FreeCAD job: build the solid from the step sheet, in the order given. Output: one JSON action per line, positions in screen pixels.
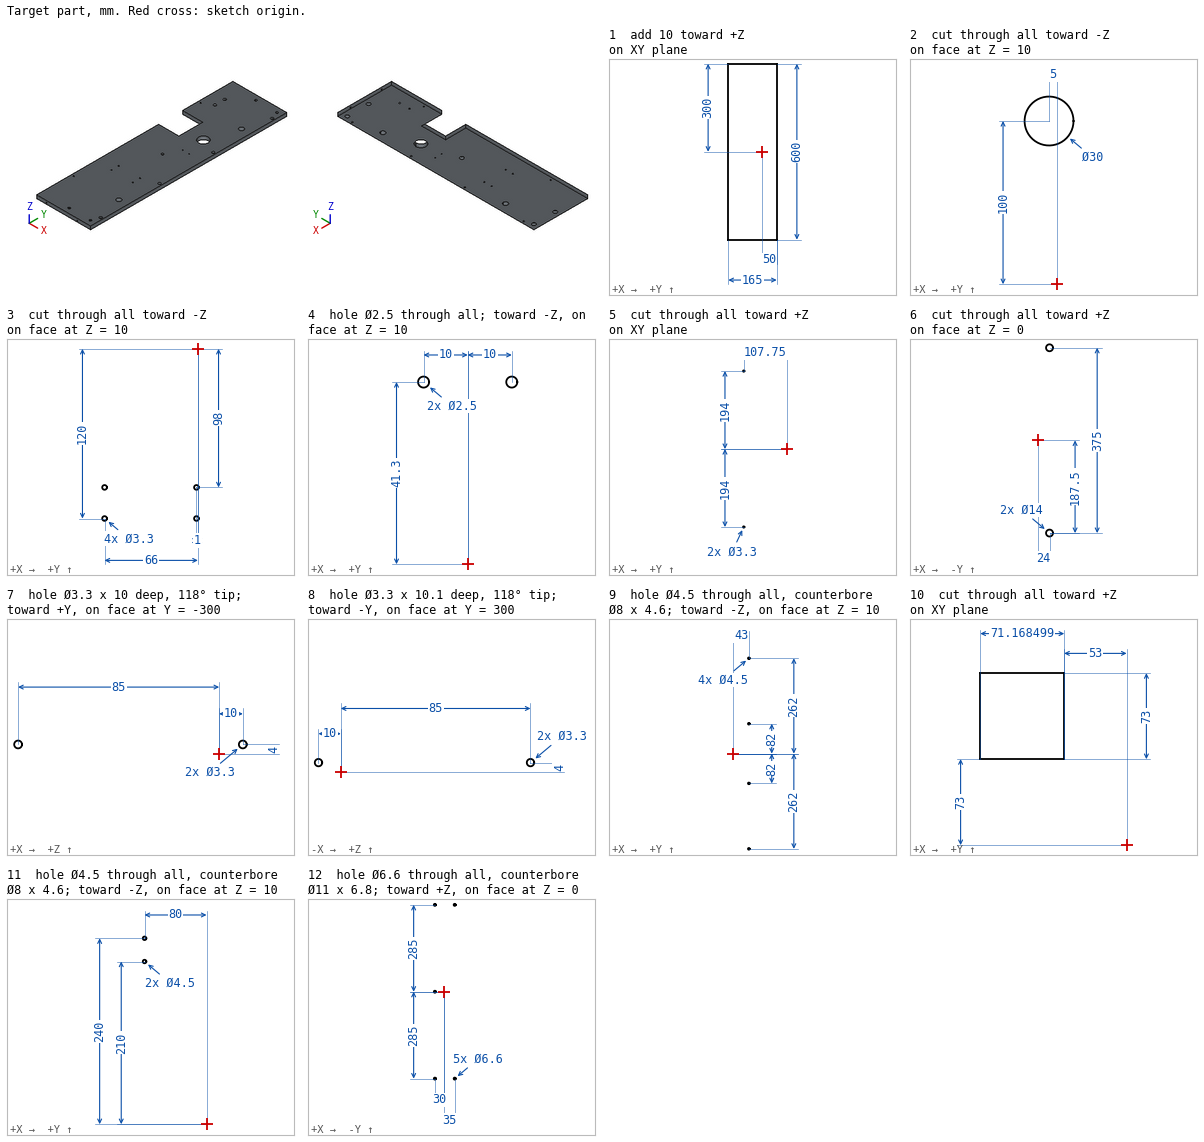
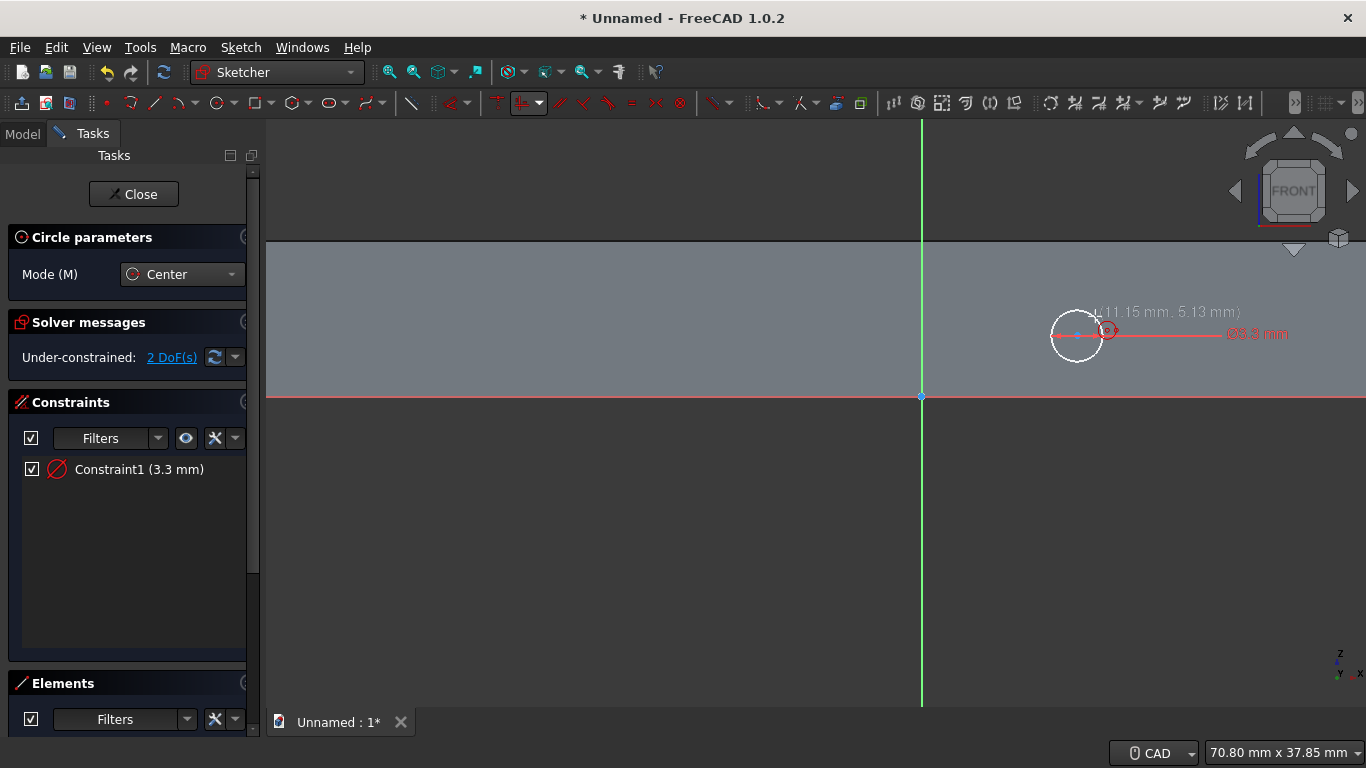
{"action": "scroll", "coordinate": [1081, 462], "scroll_direction": "down", "scroll_amount": 4}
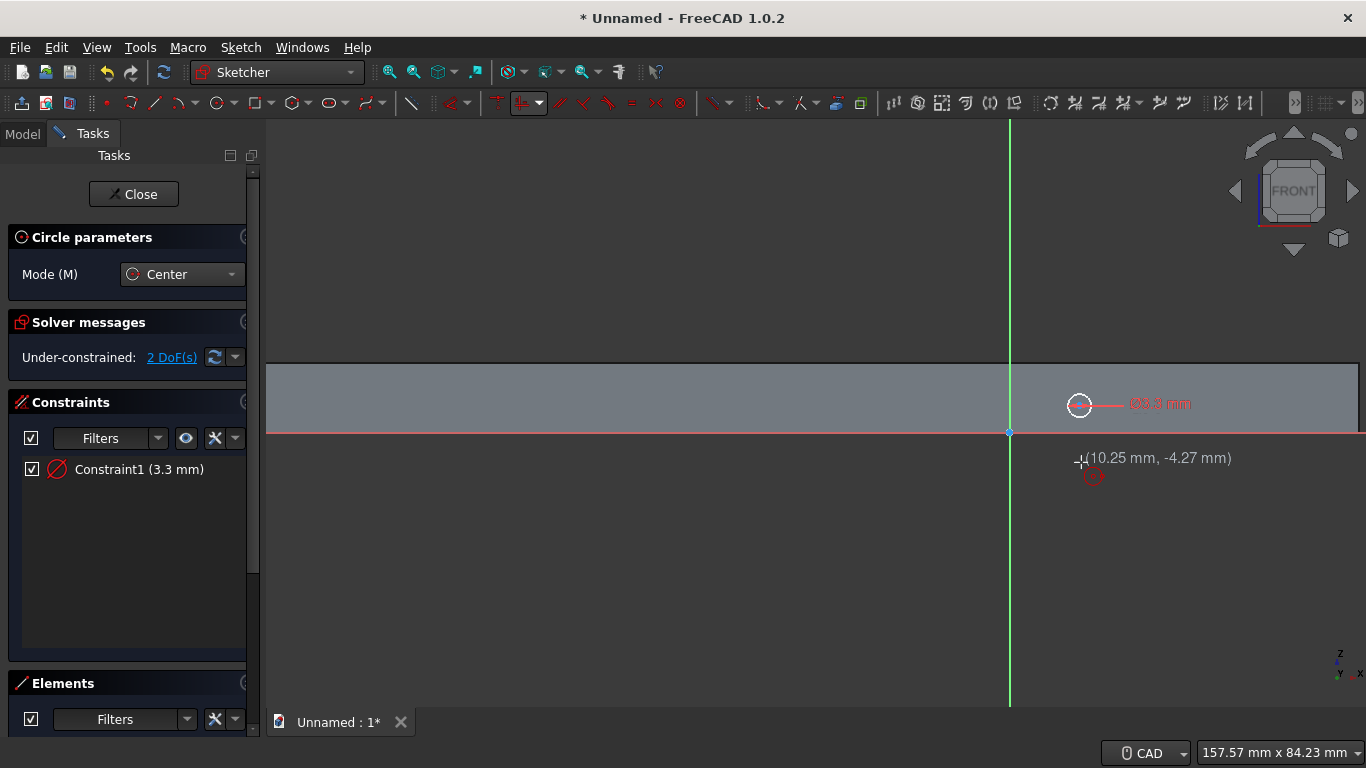
{"action": "scroll", "coordinate": [416, 405], "scroll_direction": "up", "scroll_amount": 4}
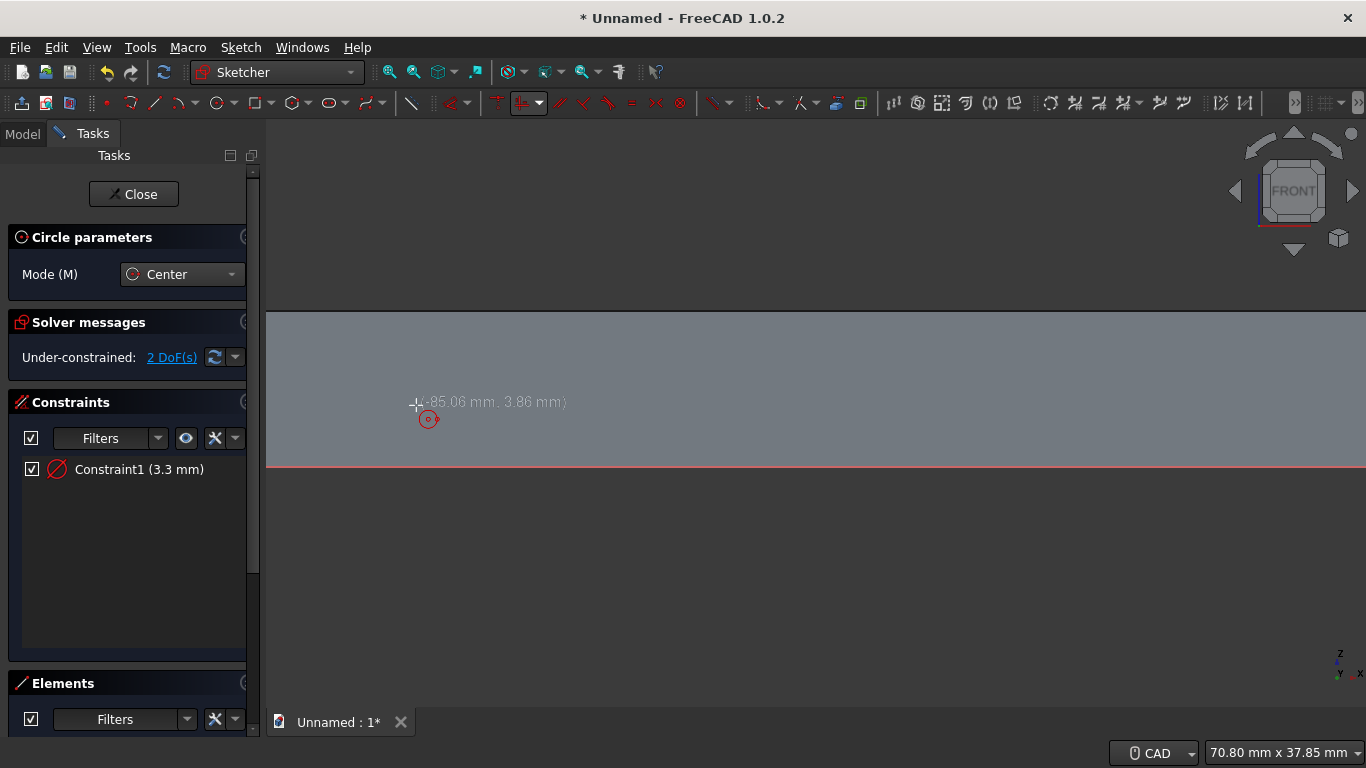
{"action": "left_click", "coordinate": [417, 404]}
{"action": "mouse_move", "coordinate": [435, 386]}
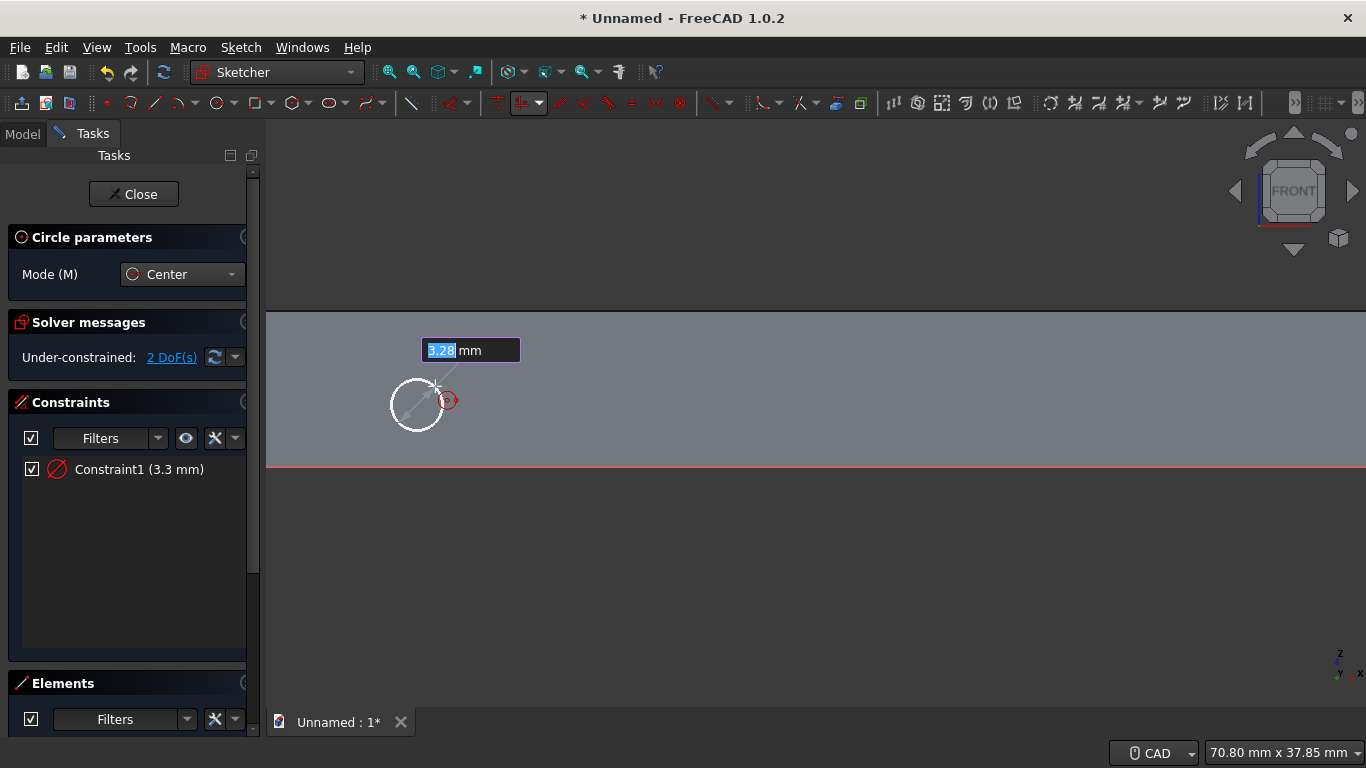
{"action": "type", "text": "3.3"}
{"action": "key", "text": "Return"}
{"action": "key", "text": "Escape"}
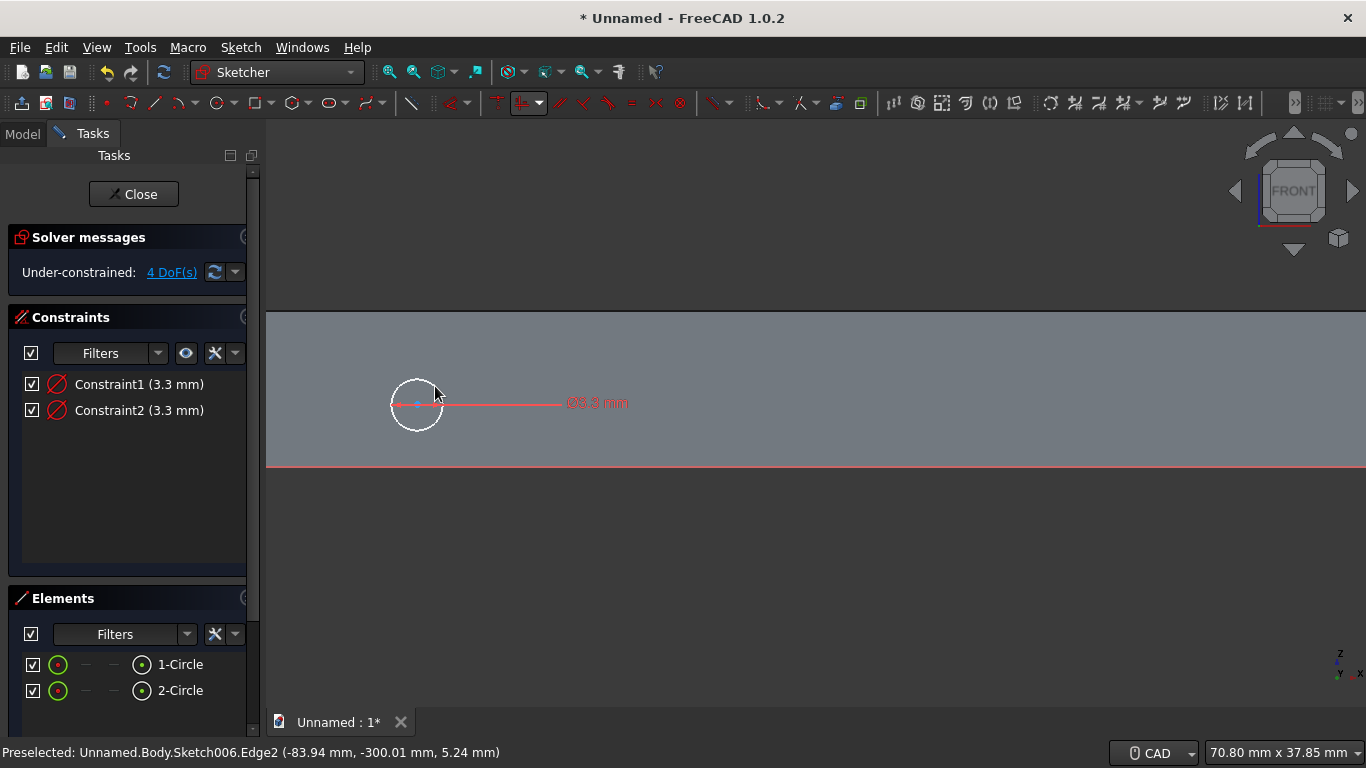
{"action": "scroll", "coordinate": [415, 405], "scroll_direction": "down", "scroll_amount": 4}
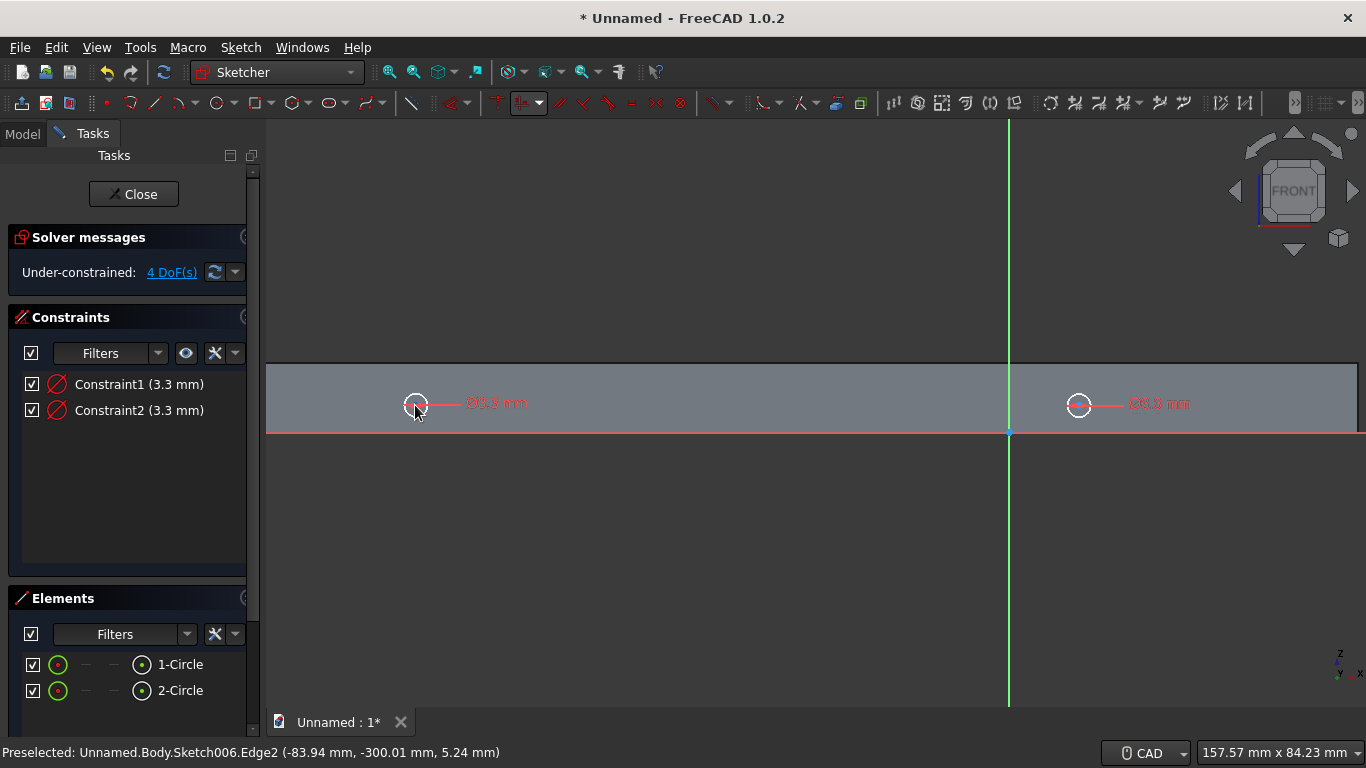
{"action": "left_click", "coordinate": [1079, 406]}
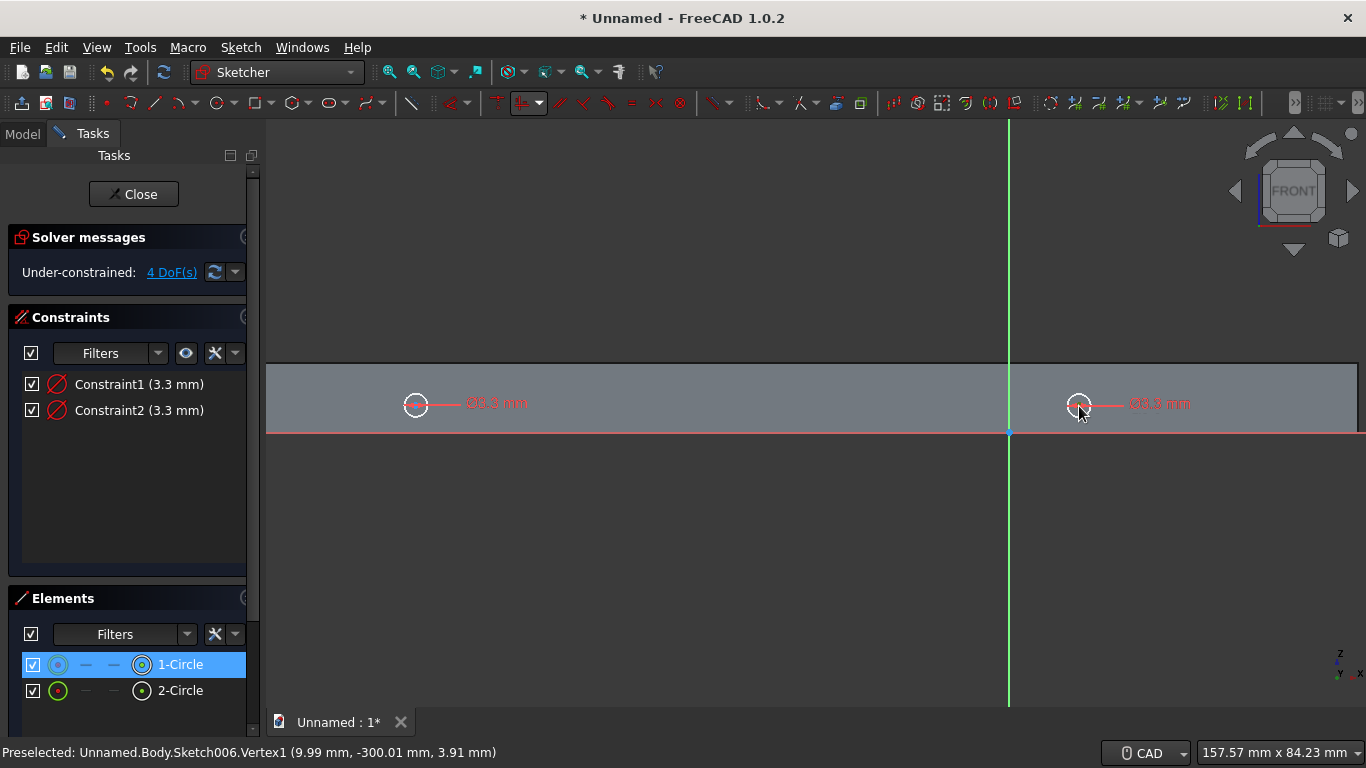
{"action": "left_click", "coordinate": [416, 405]}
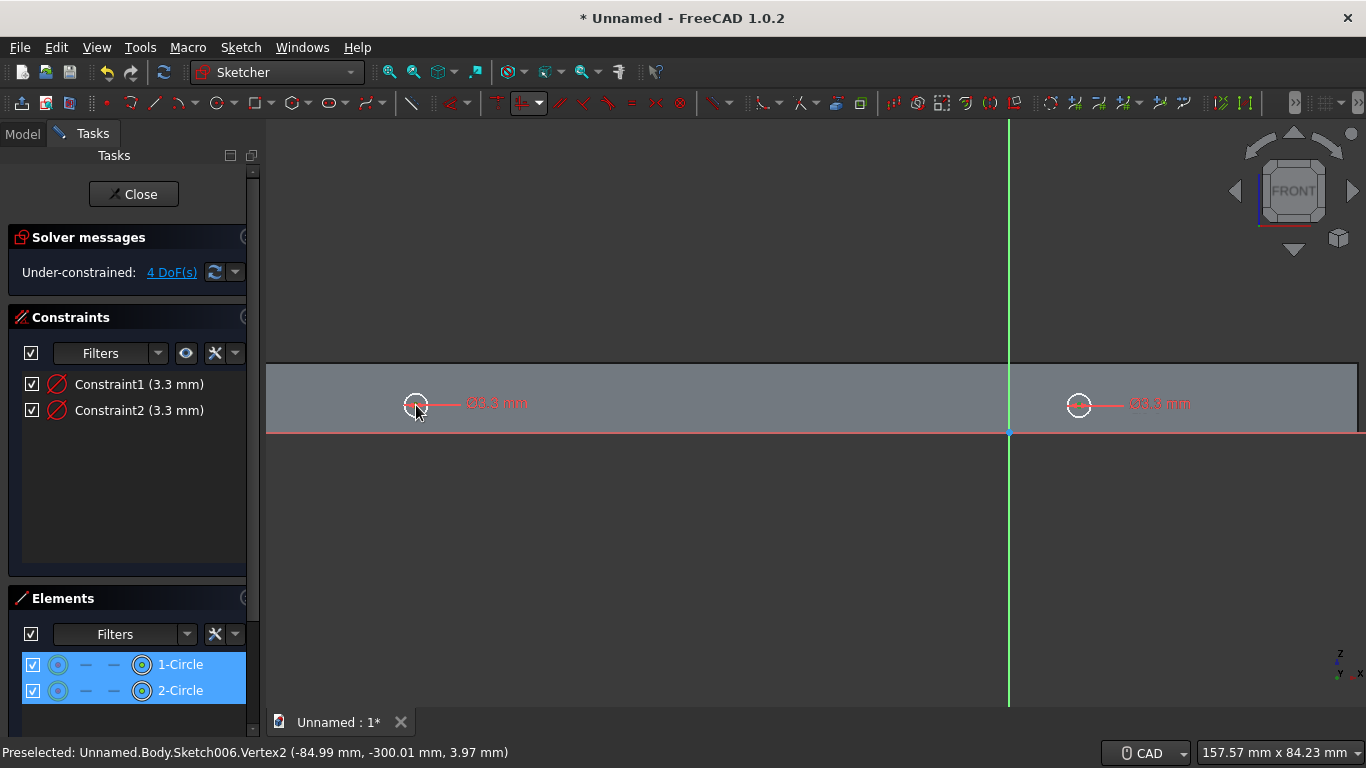
{"action": "left_click", "coordinate": [542, 104]}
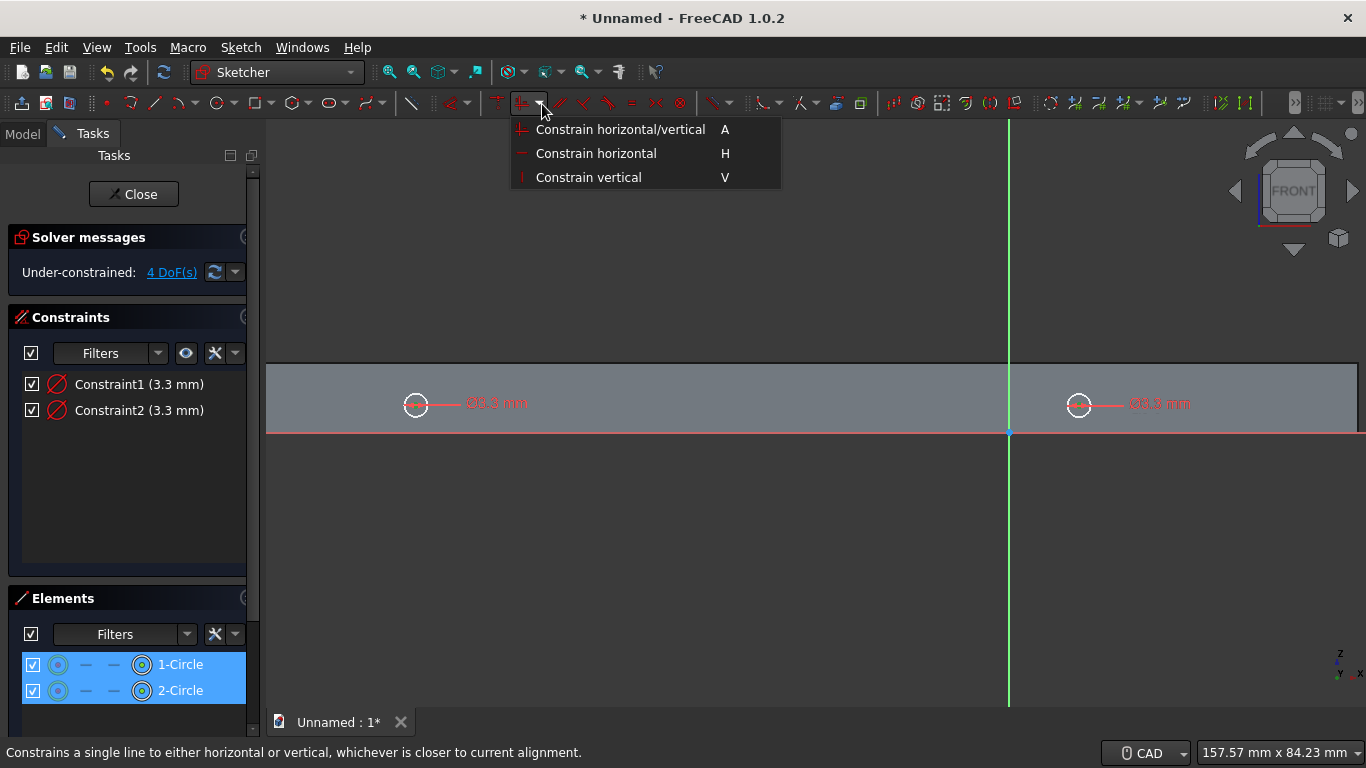
{"action": "left_click", "coordinate": [646, 153]}